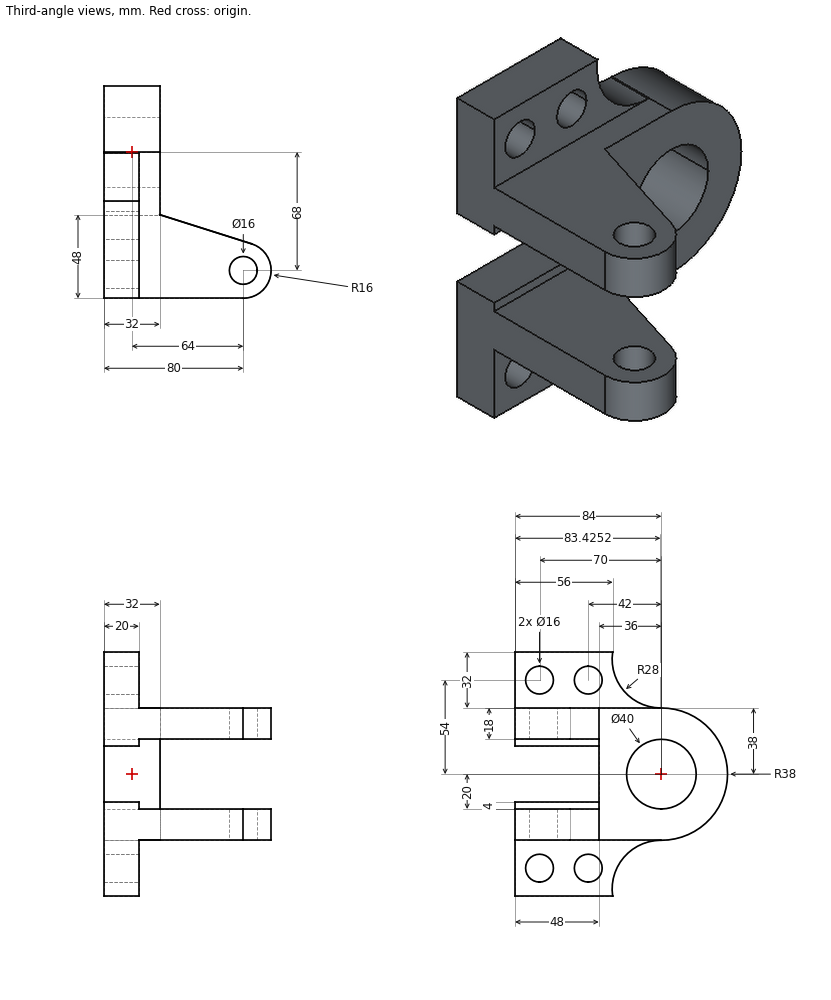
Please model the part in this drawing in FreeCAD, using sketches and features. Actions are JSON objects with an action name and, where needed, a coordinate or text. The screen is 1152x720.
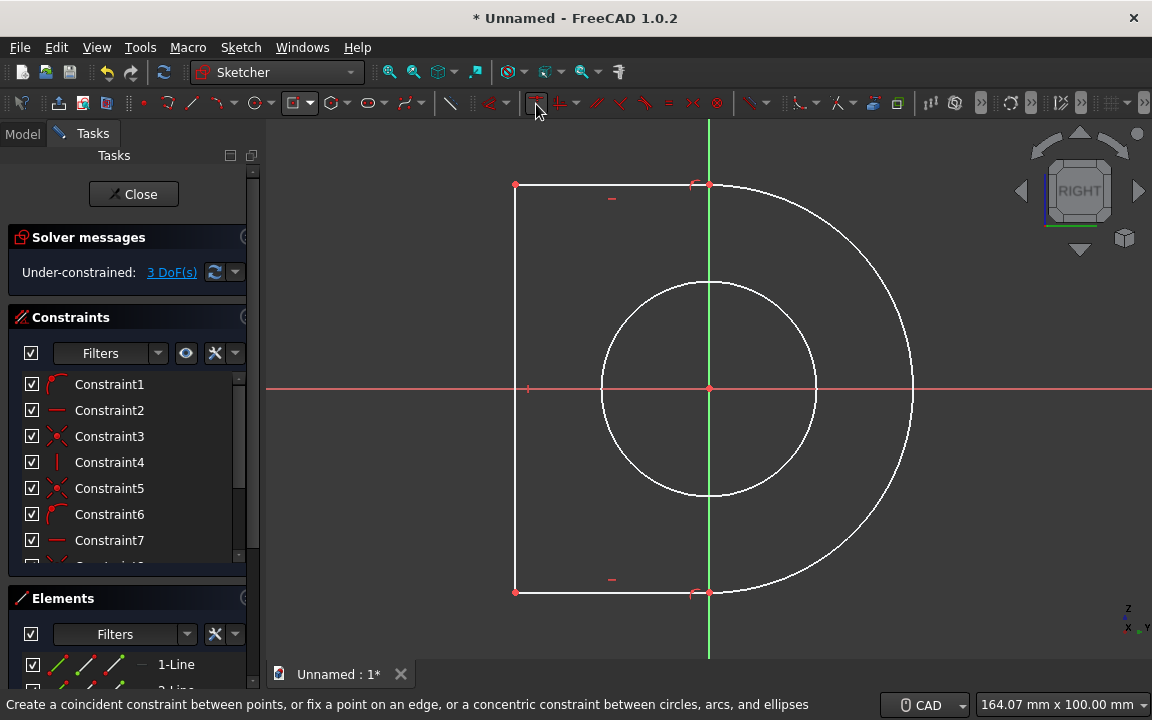
{"action": "left_click", "coordinate": [490, 104]}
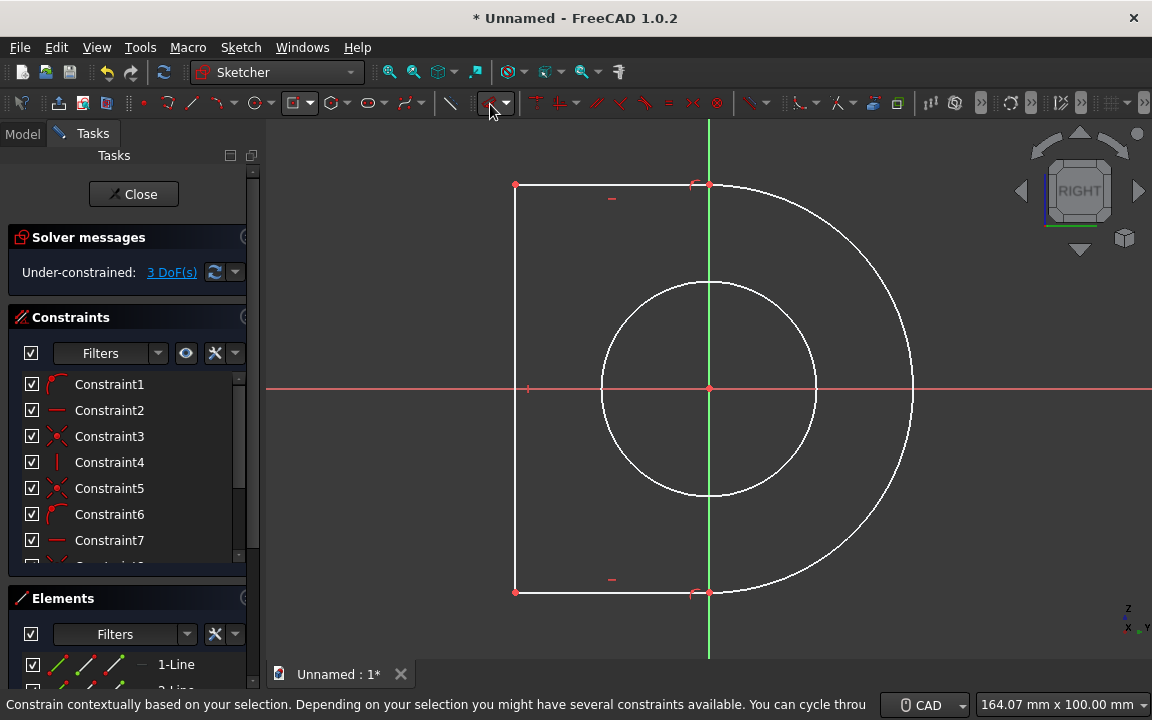
{"action": "left_click", "coordinate": [874, 509]}
{"action": "left_click", "coordinate": [900, 528]}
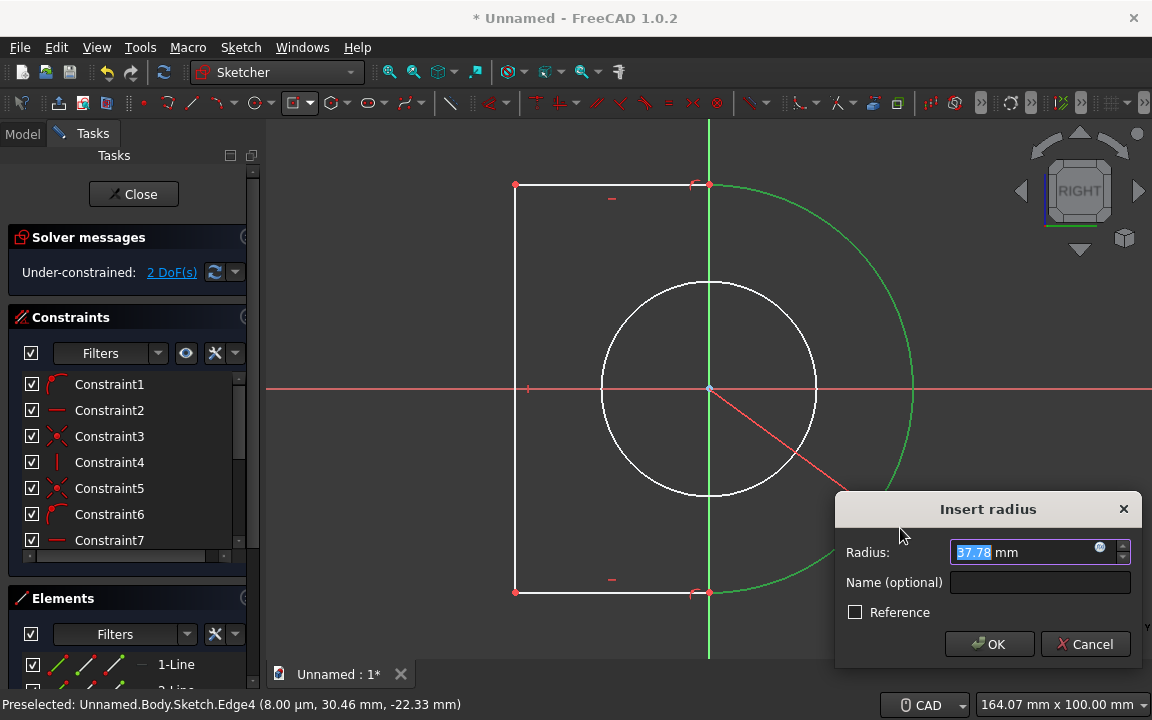
{"action": "type", "text": "38"}
{"action": "key", "text": "Return"}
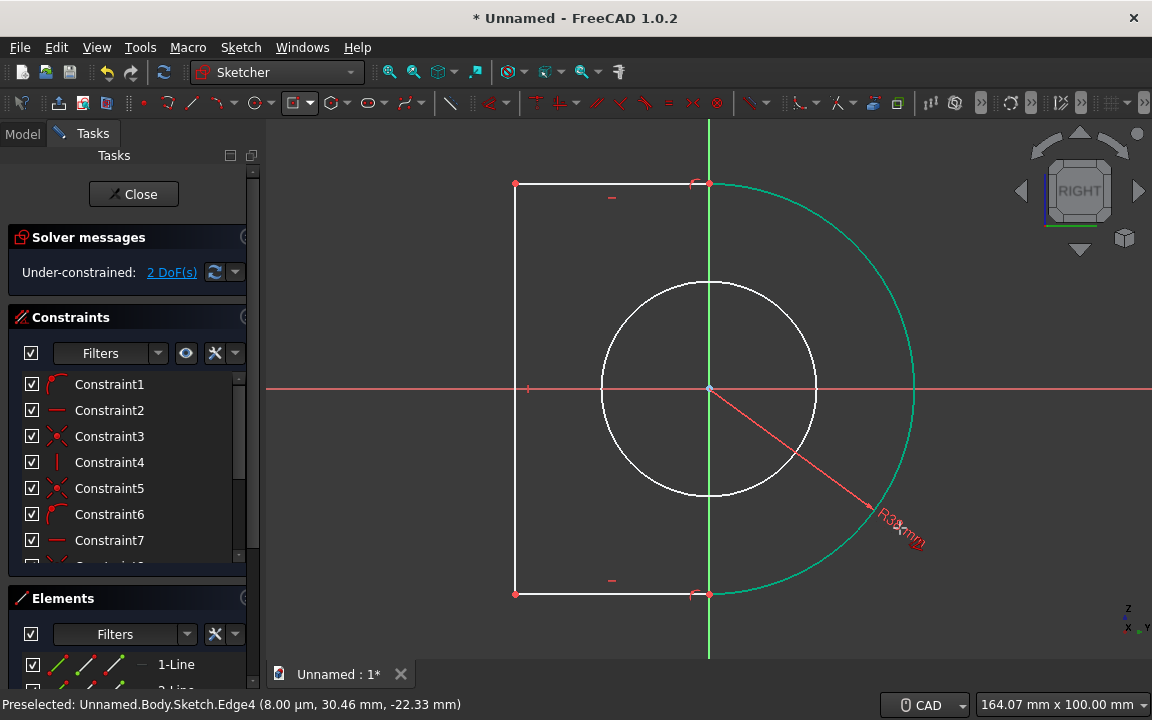
{"action": "left_click", "coordinate": [785, 313]}
{"action": "left_click", "coordinate": [808, 290]}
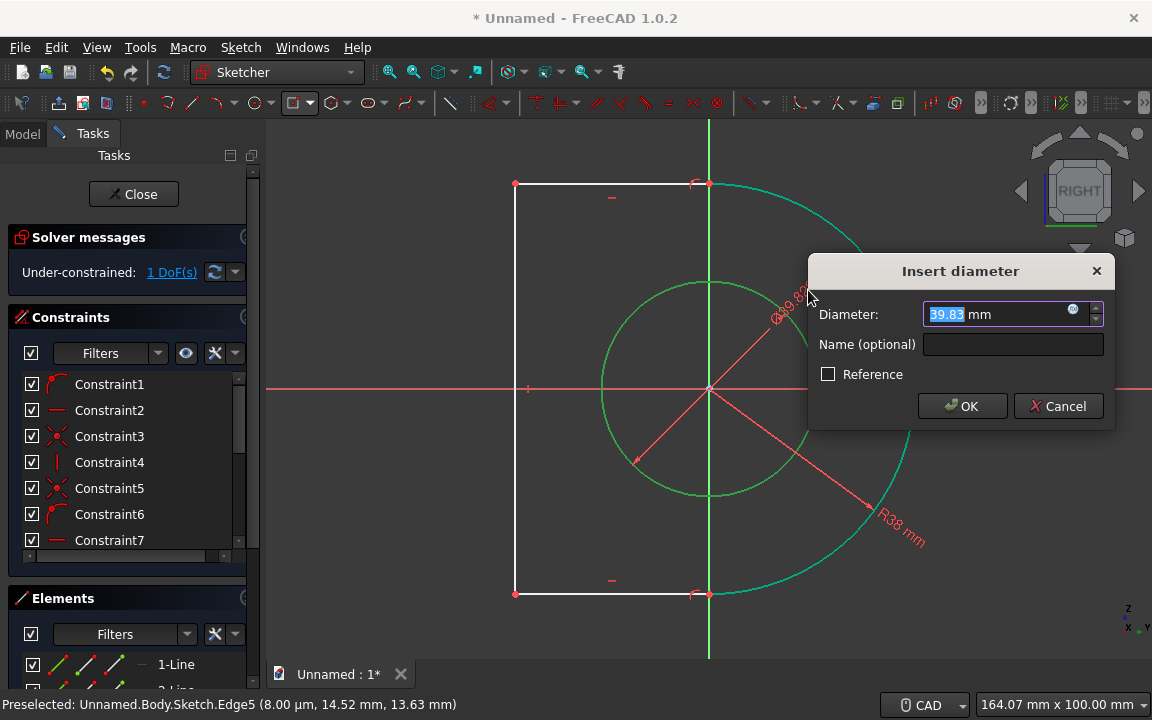
{"action": "type", "text": "40"}
{"action": "key", "text": "Return"}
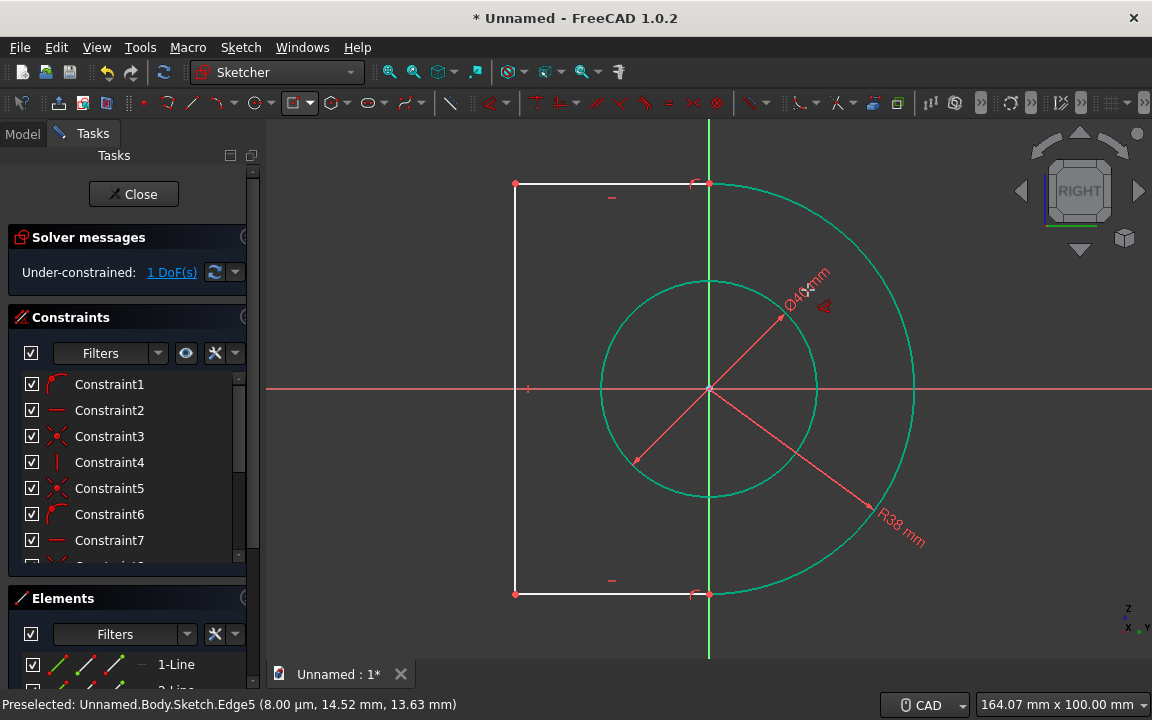
{"action": "left_click", "coordinate": [651, 184]}
{"action": "left_click", "coordinate": [612, 150]}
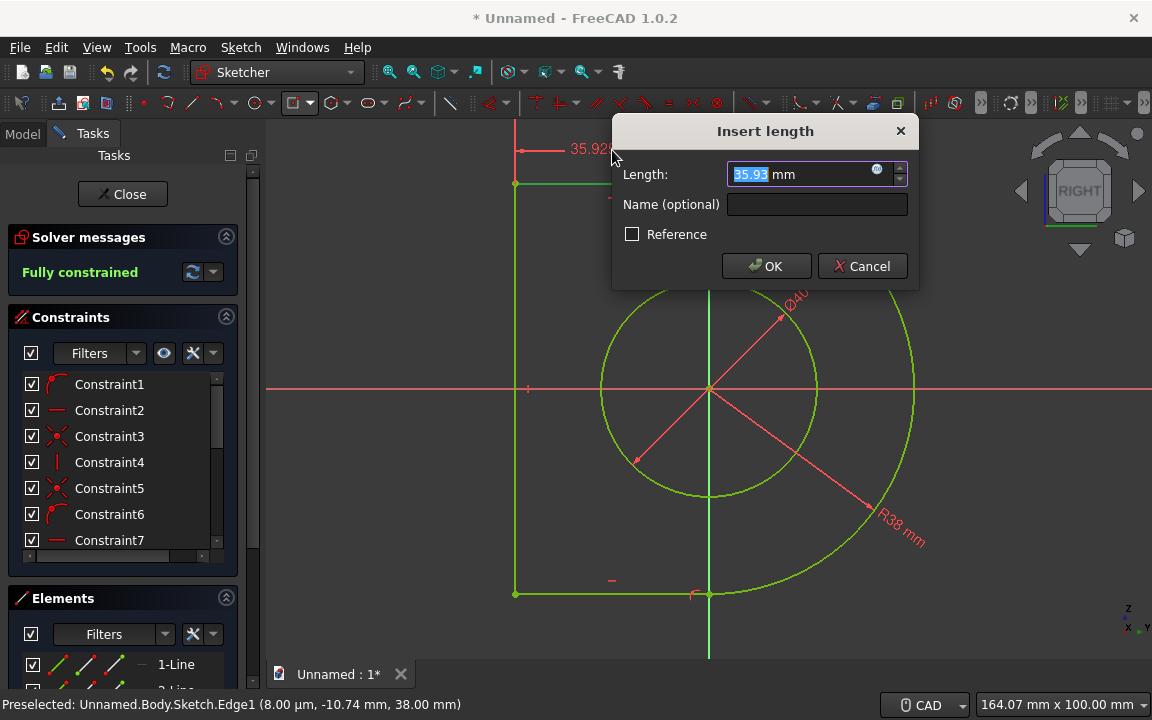
{"action": "type", "text": "36"}
{"action": "key", "text": "Return"}
{"action": "key", "text": "Escape"}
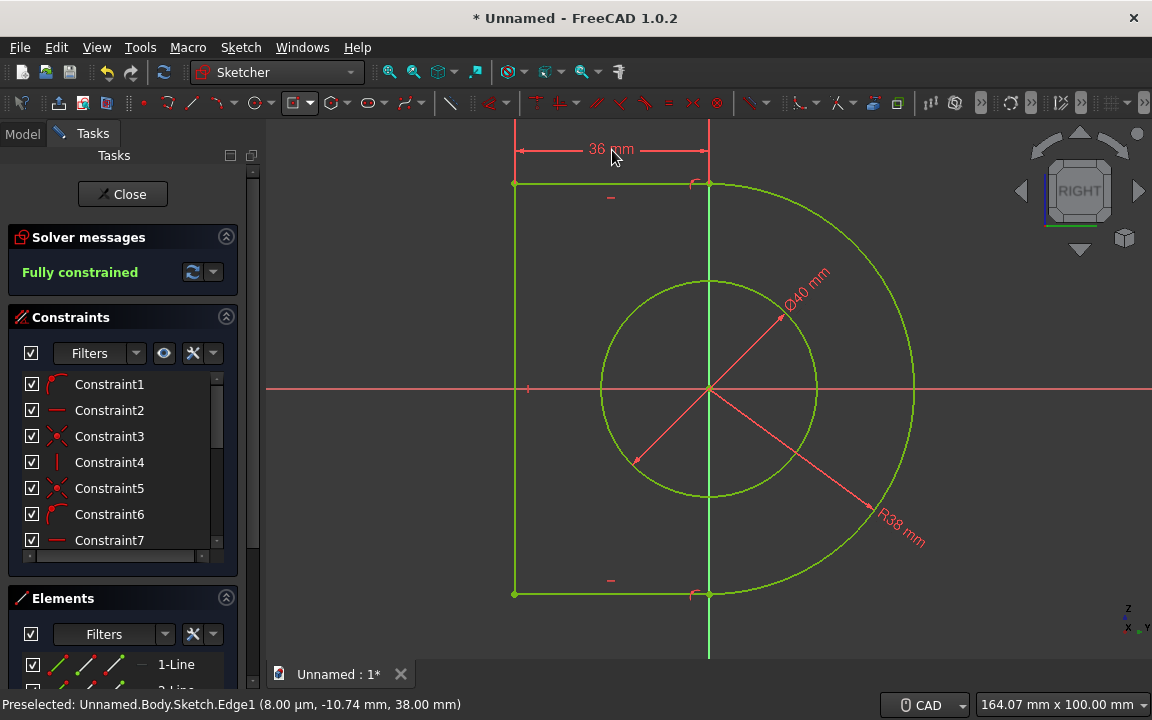
{"action": "left_click", "coordinate": [123, 194]}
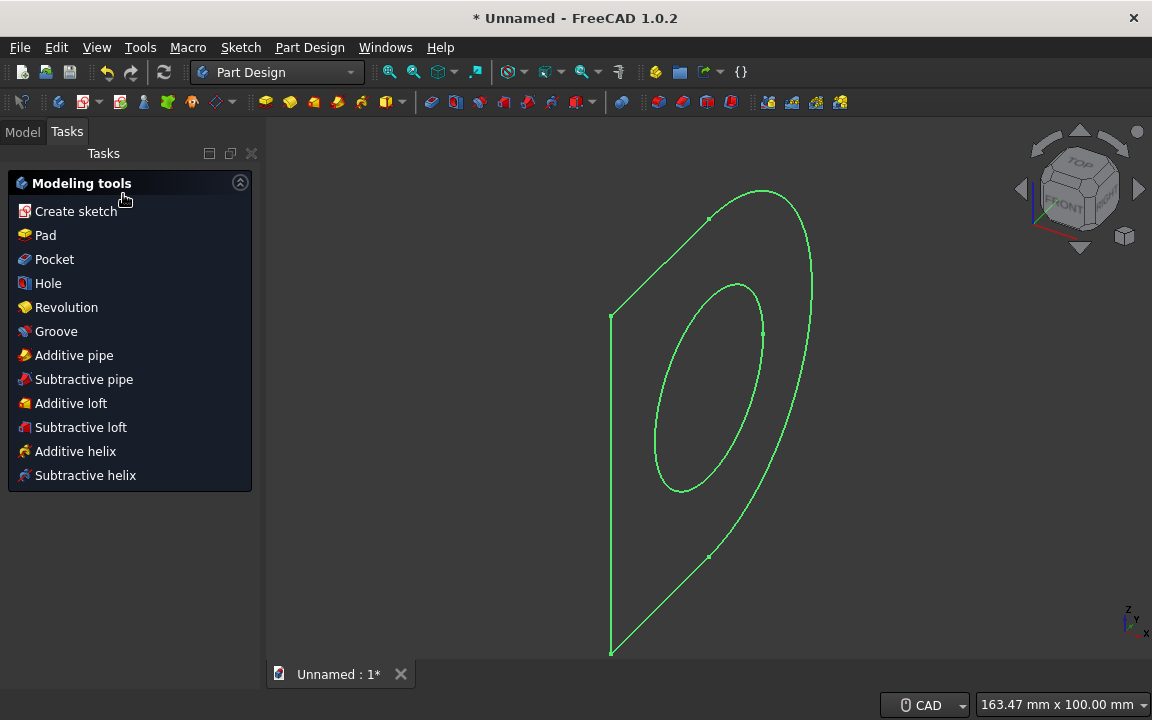
{"action": "left_click", "coordinate": [266, 102]}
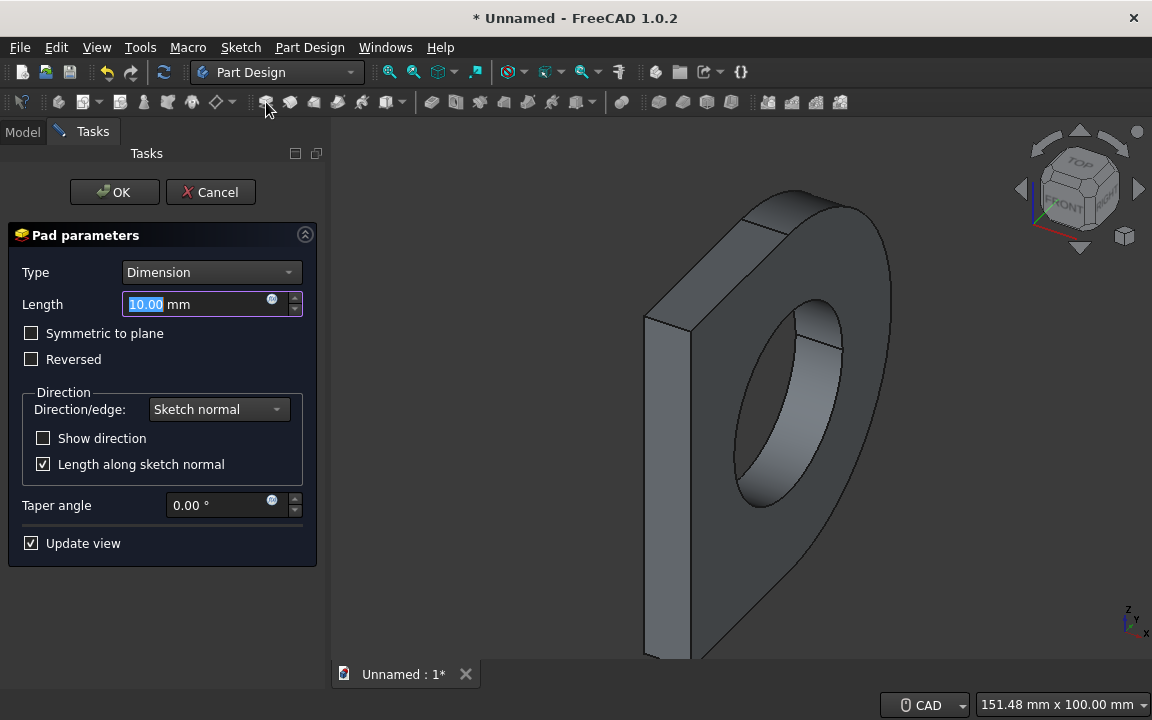
{"action": "type", "text": "32"}
{"action": "key", "text": "Tab"}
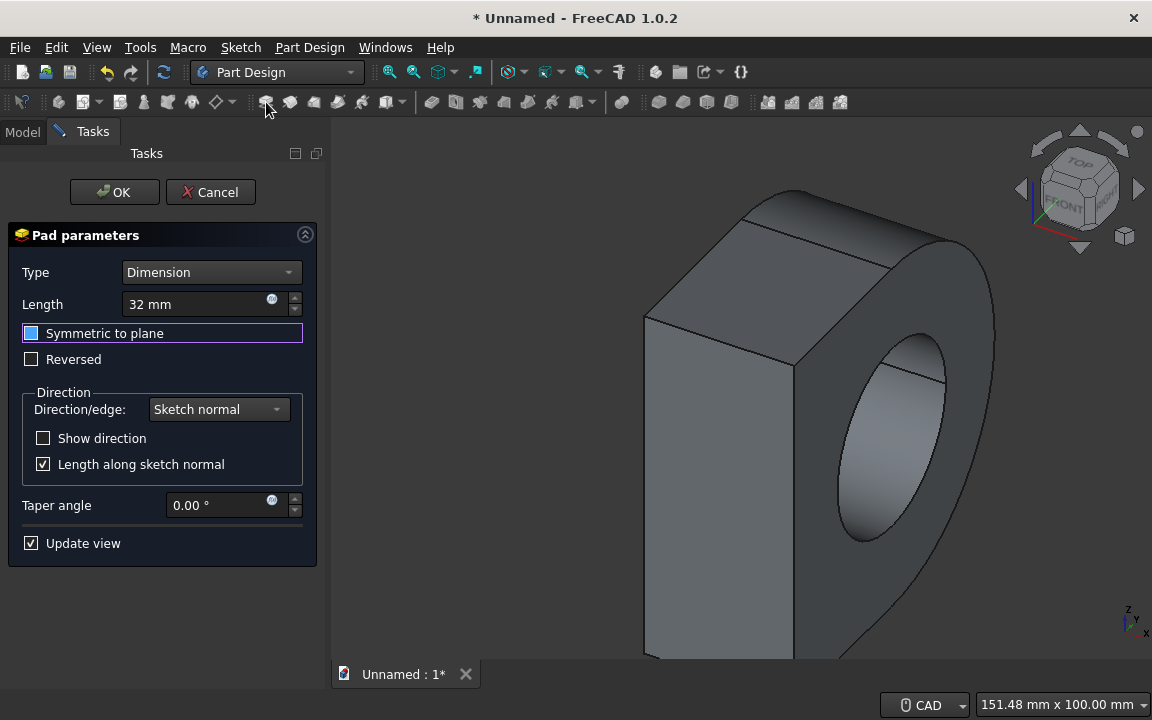
{"action": "left_click", "coordinate": [30, 333]}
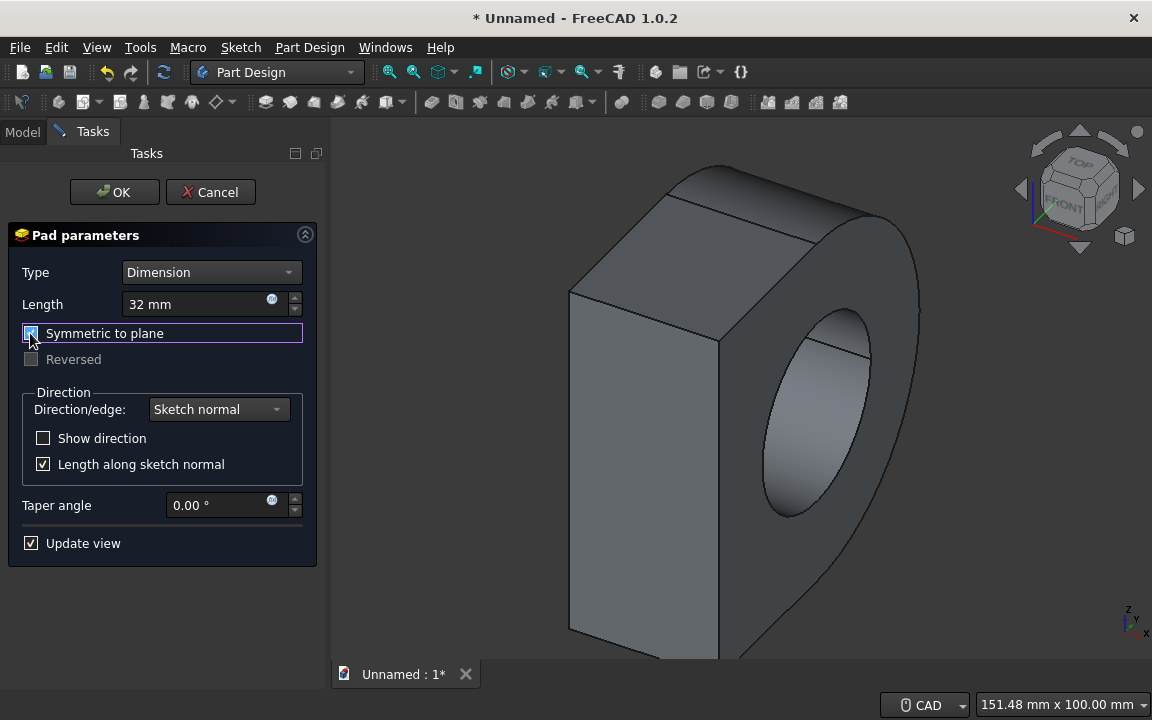
{"action": "left_click", "coordinate": [115, 192]}